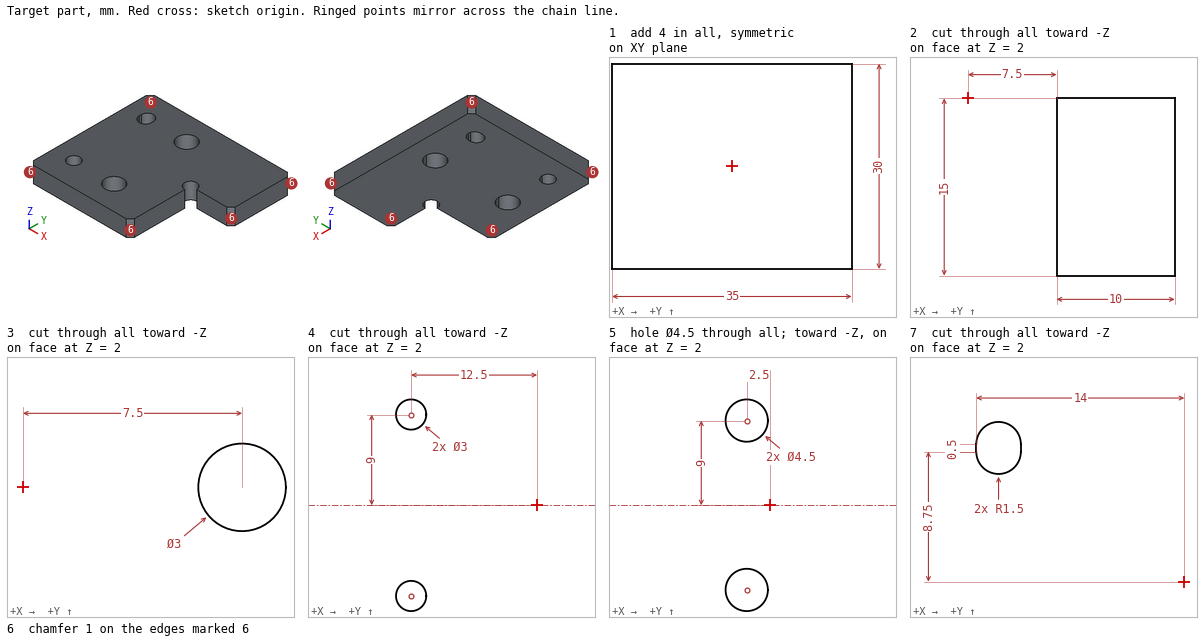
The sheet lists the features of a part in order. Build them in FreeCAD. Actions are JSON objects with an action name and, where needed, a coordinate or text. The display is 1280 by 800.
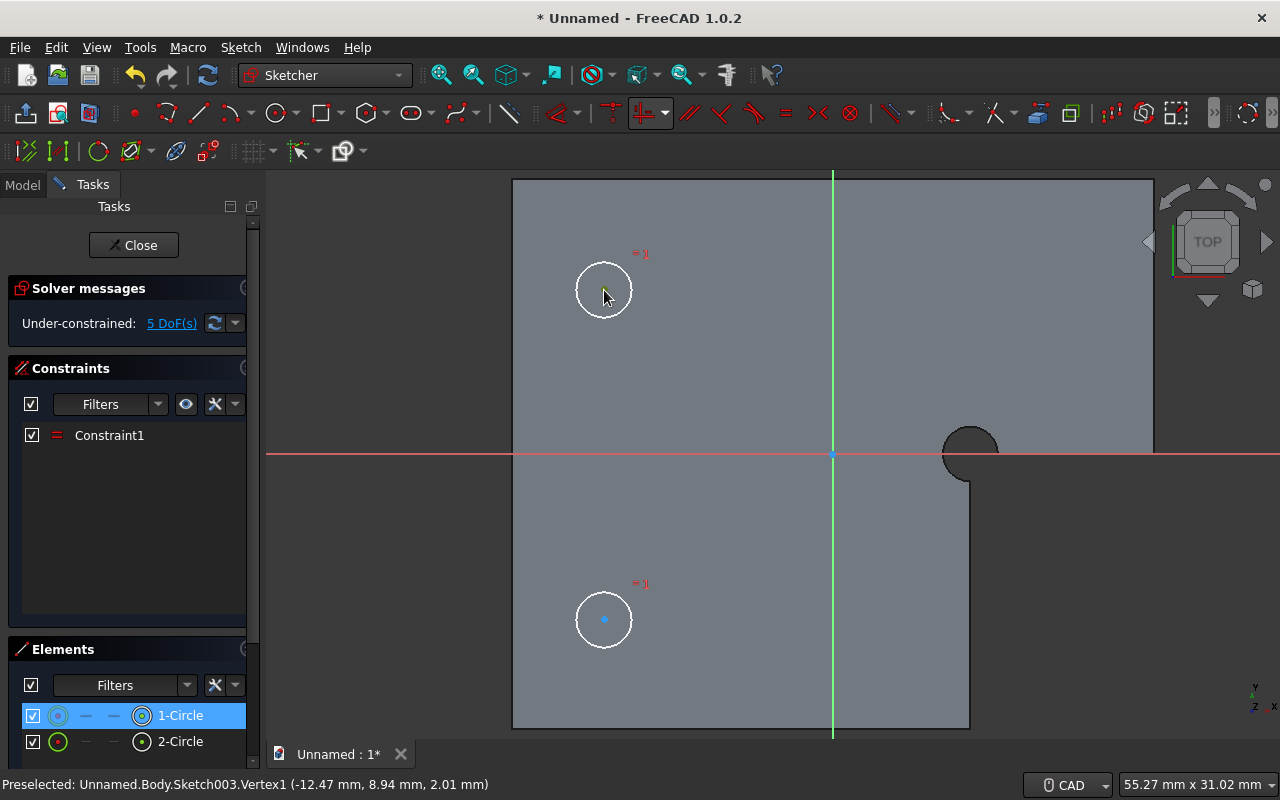
{"action": "left_click", "coordinate": [604, 620]}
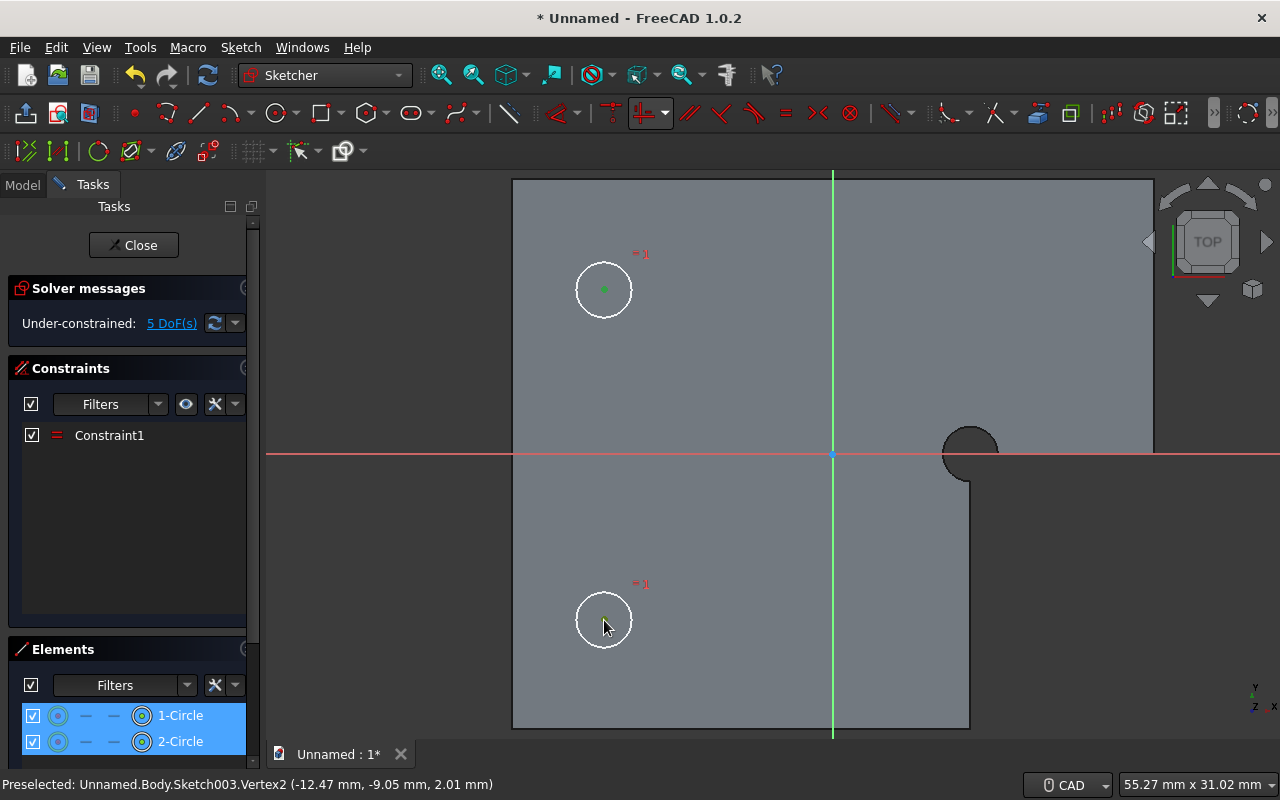
{"action": "left_click", "coordinate": [353, 454]}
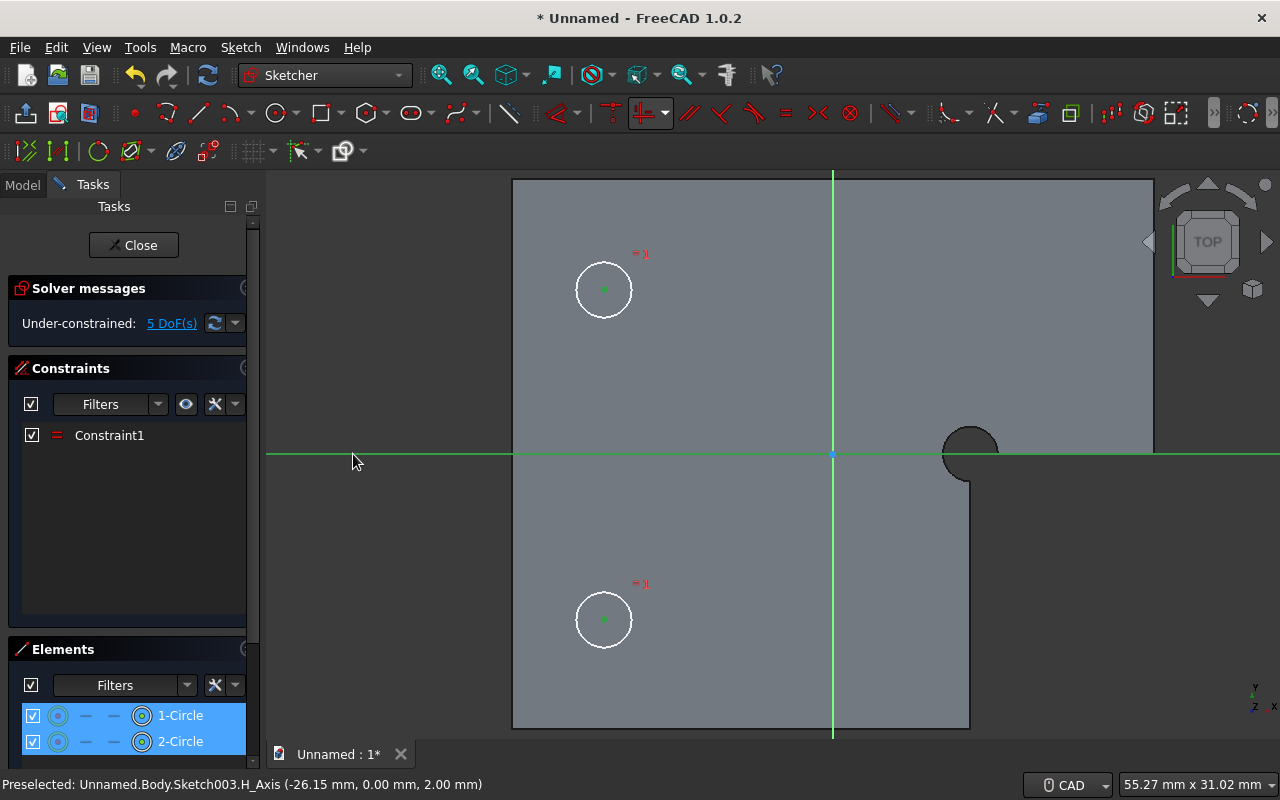
{"action": "key", "text": "s"}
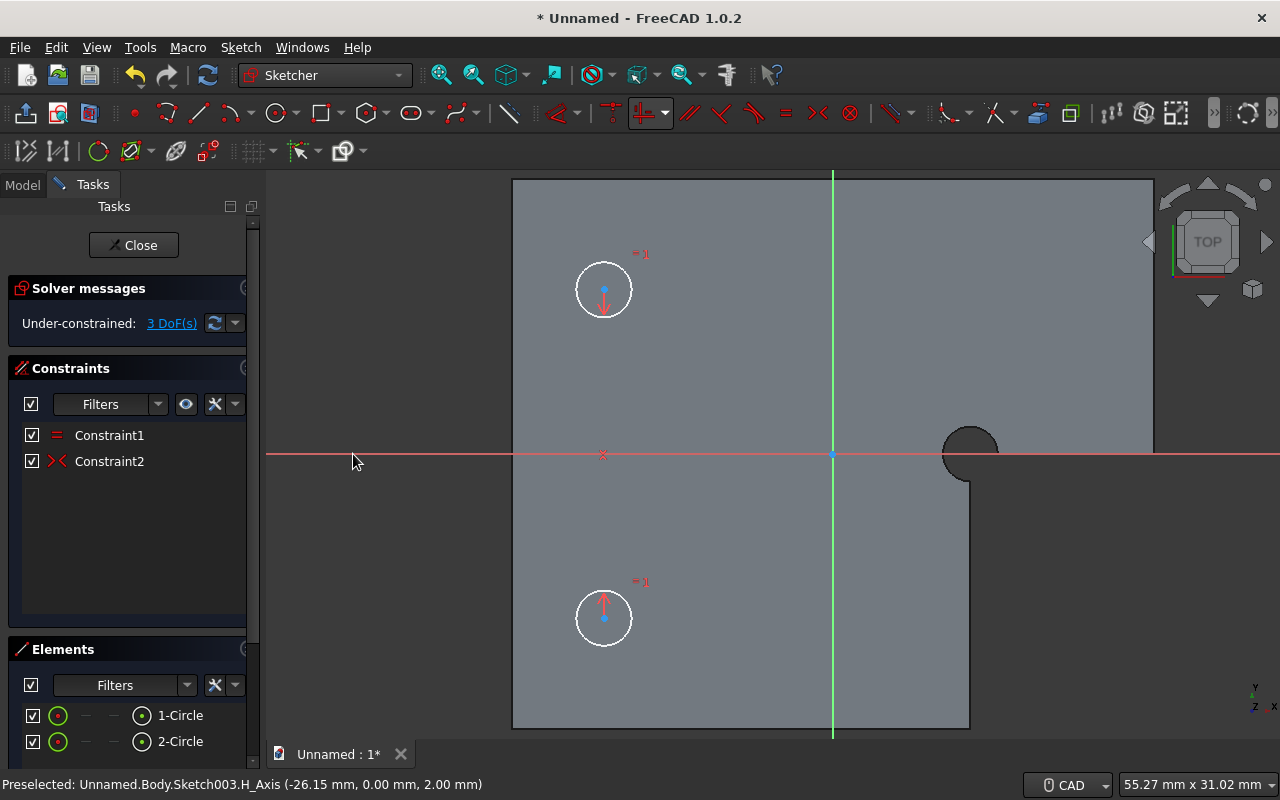
{"action": "key", "text": "d"}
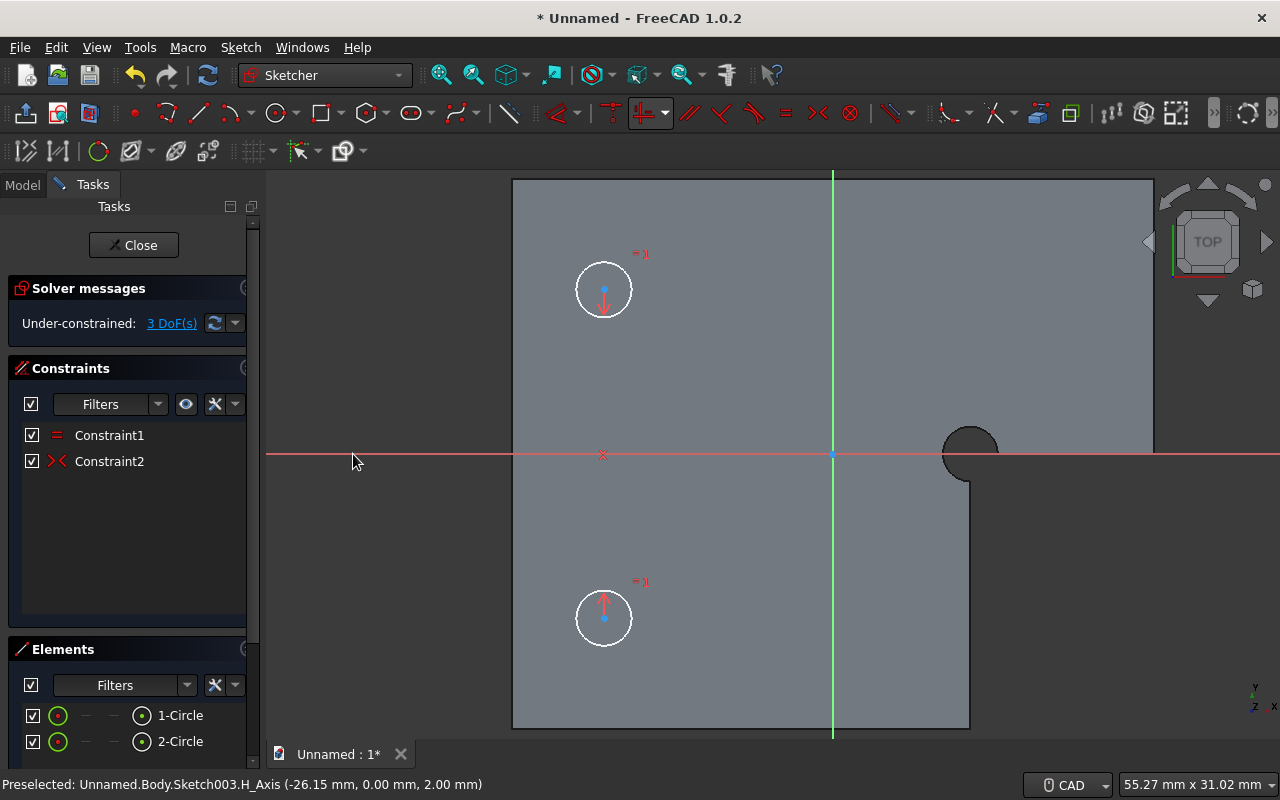
{"action": "left_click", "coordinate": [623, 270]}
{"action": "left_click", "coordinate": [645, 247]}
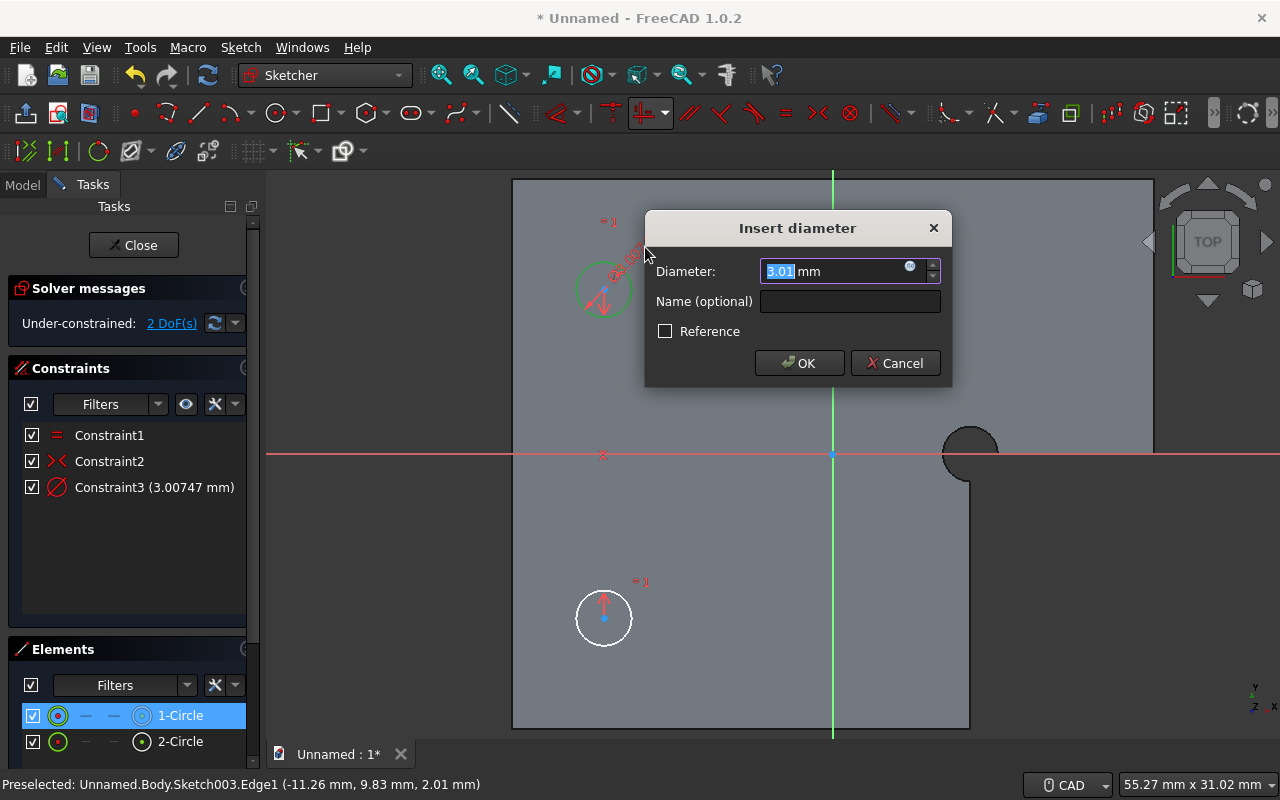
{"action": "type", "text": "3"}
{"action": "key", "text": "Return"}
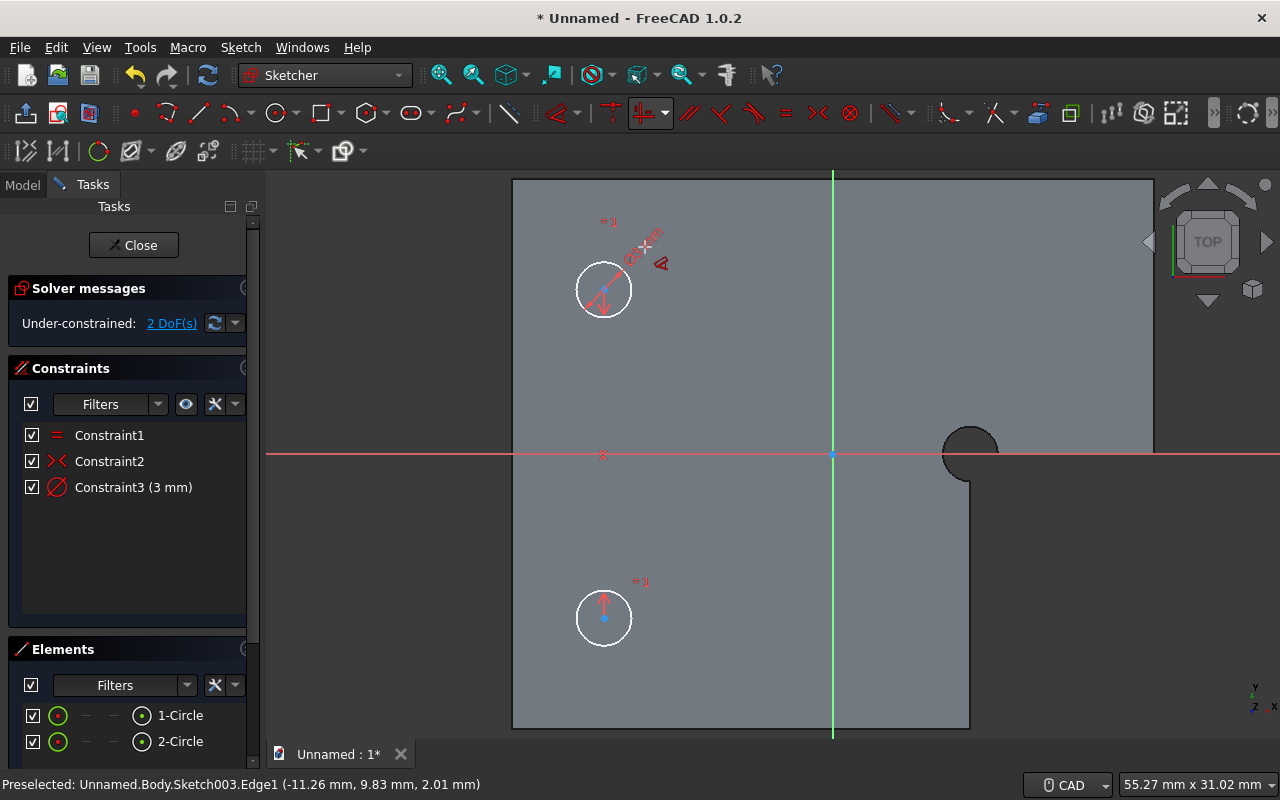
{"action": "left_click", "coordinate": [604, 290]}
{"action": "left_click", "coordinate": [867, 372]}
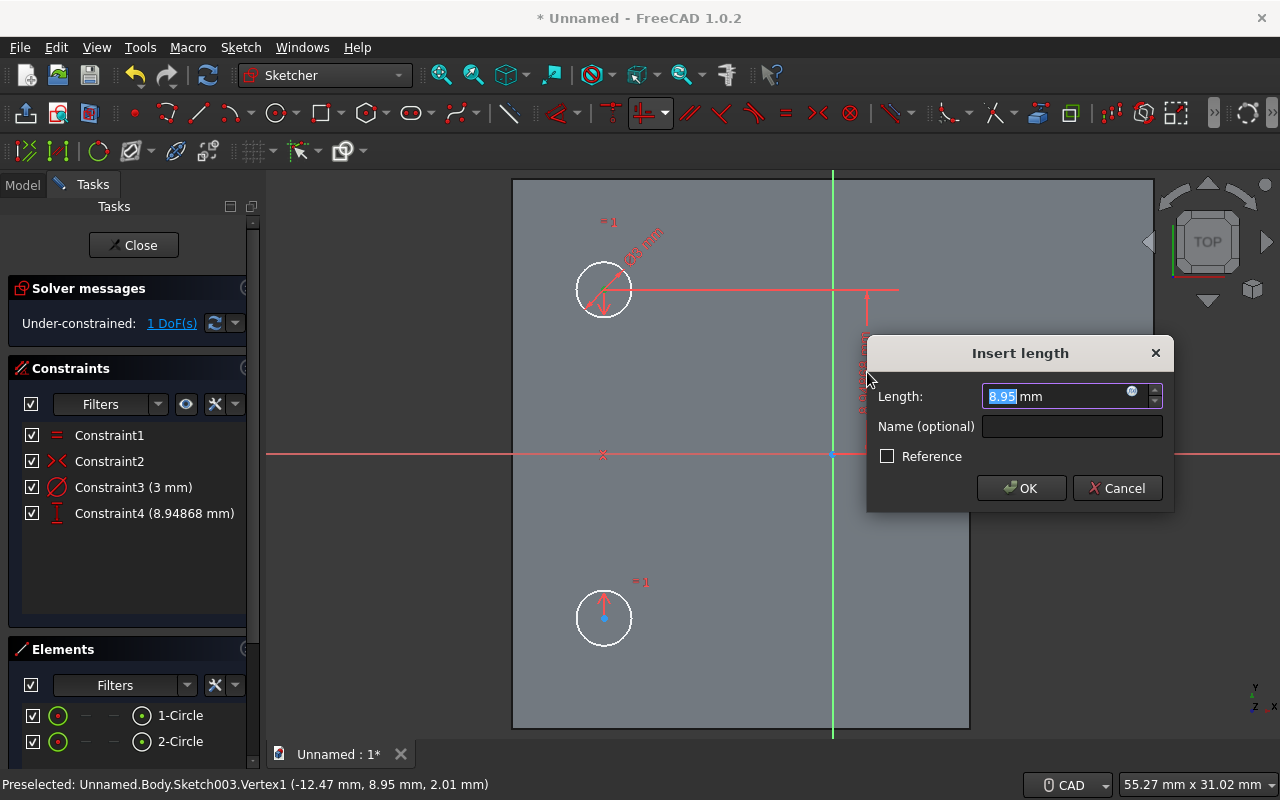
{"action": "type", "text": "9"}
{"action": "key", "text": "Return"}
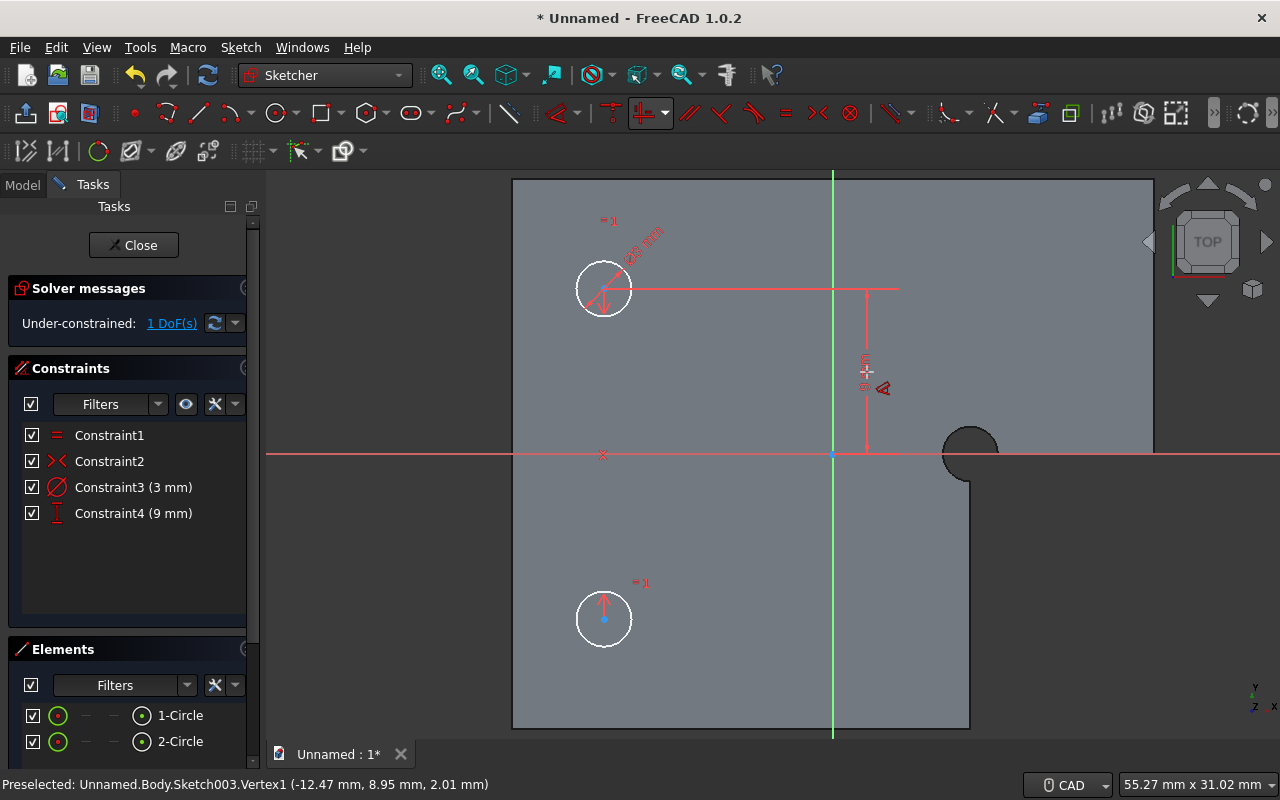
{"action": "left_click", "coordinate": [604, 289]}
{"action": "left_click", "coordinate": [718, 255]}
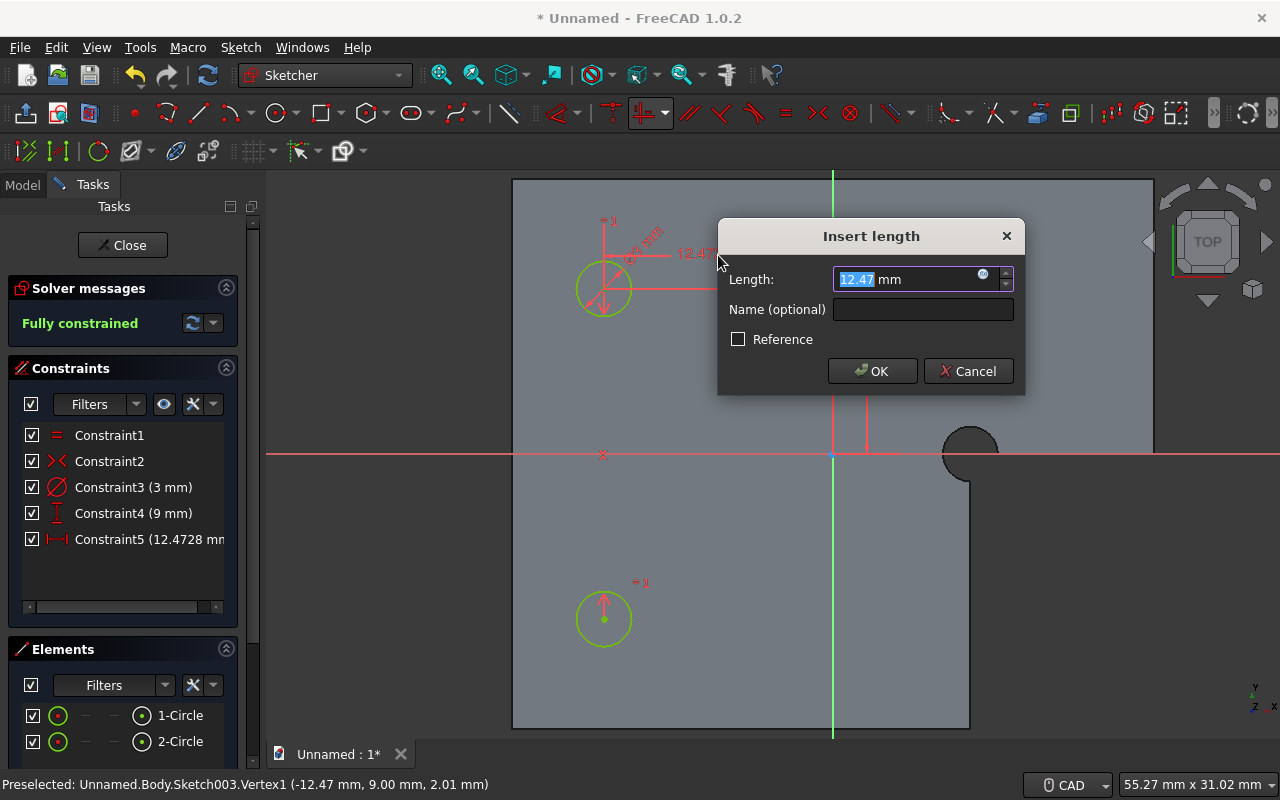
{"action": "type", "text": "12.5"}
{"action": "key", "text": "Return"}
{"action": "key", "text": "Escape"}